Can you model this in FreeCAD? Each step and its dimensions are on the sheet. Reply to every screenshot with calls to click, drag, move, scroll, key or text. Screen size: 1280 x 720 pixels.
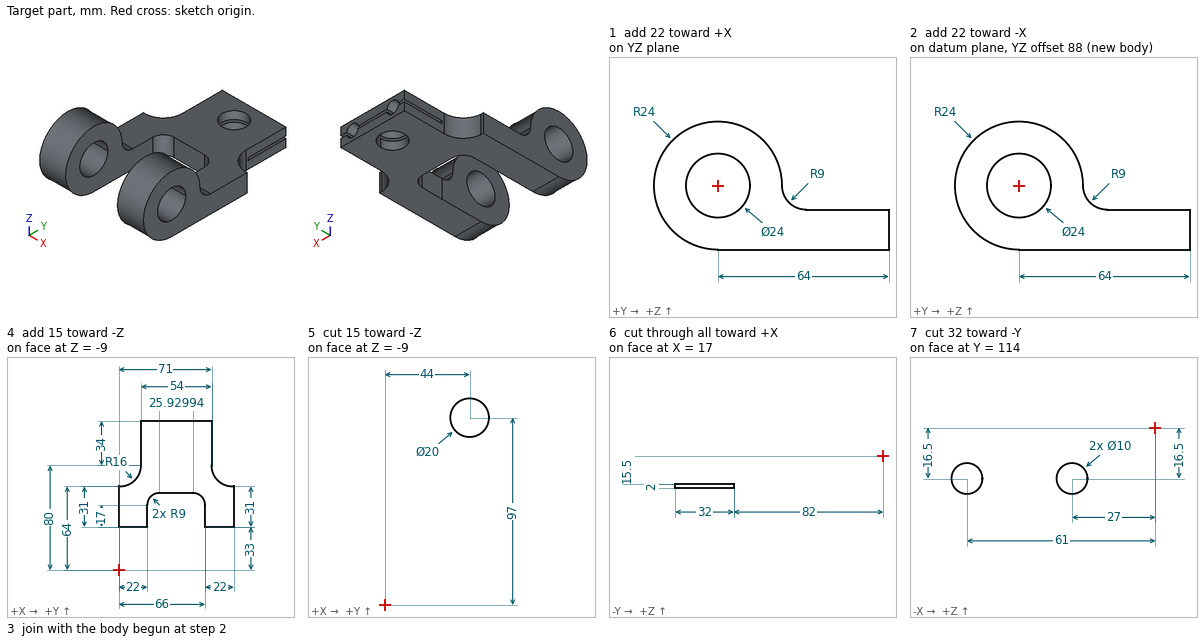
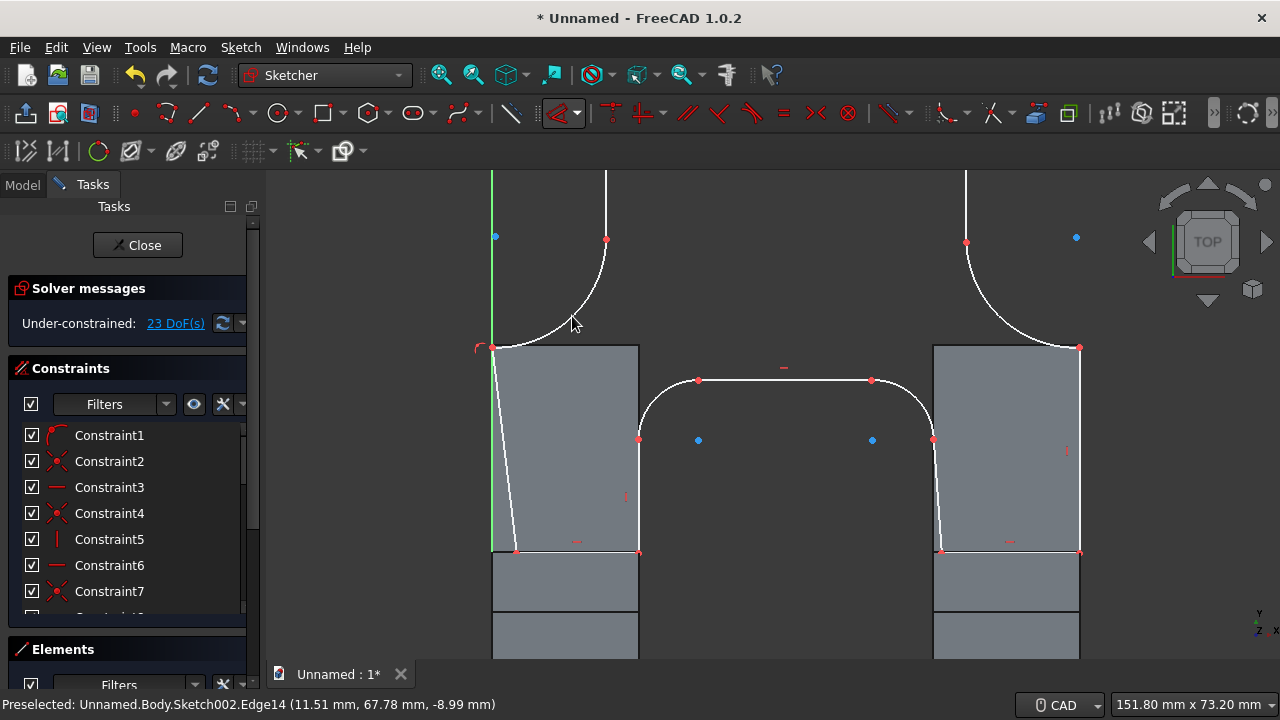
click(639, 519)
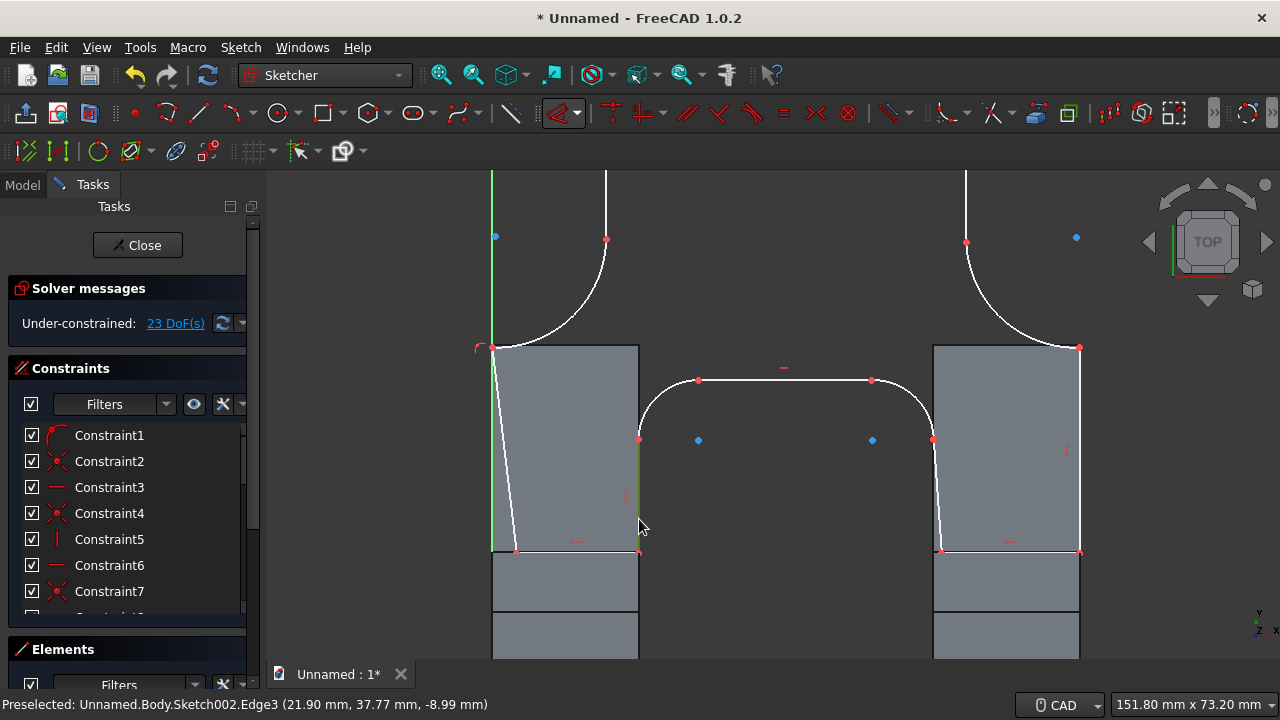
click(671, 387)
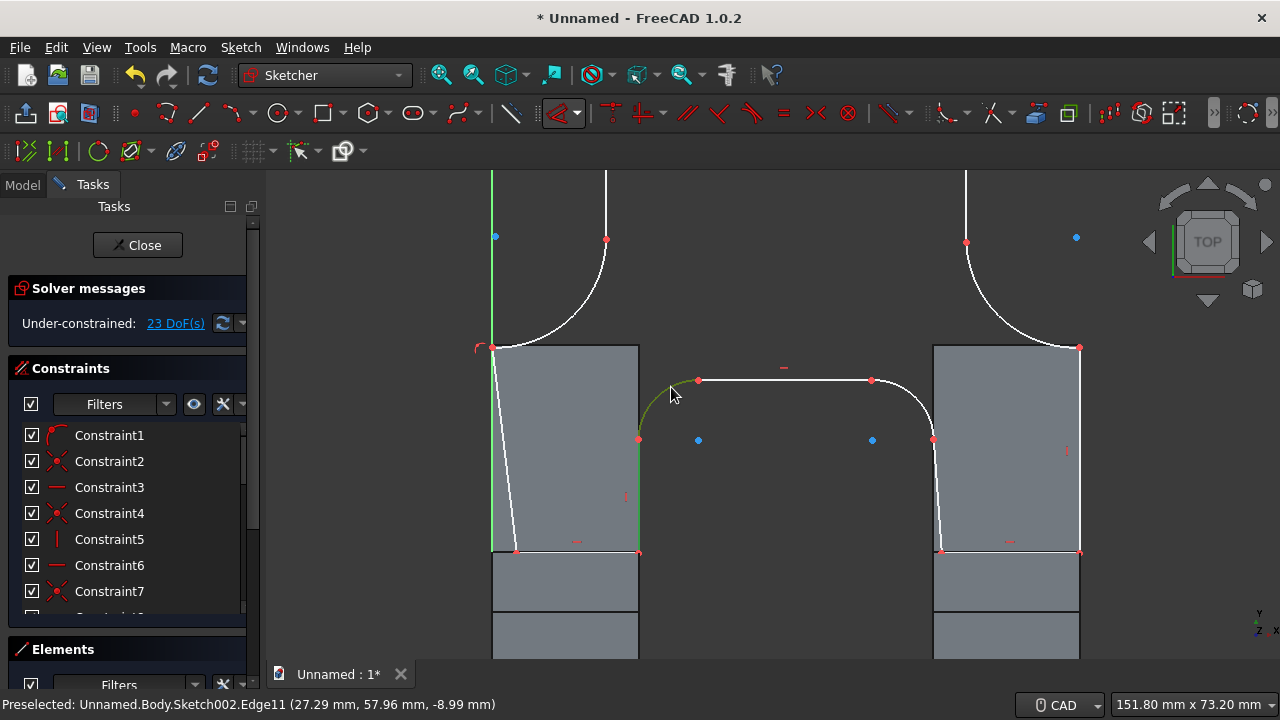
click(752, 114)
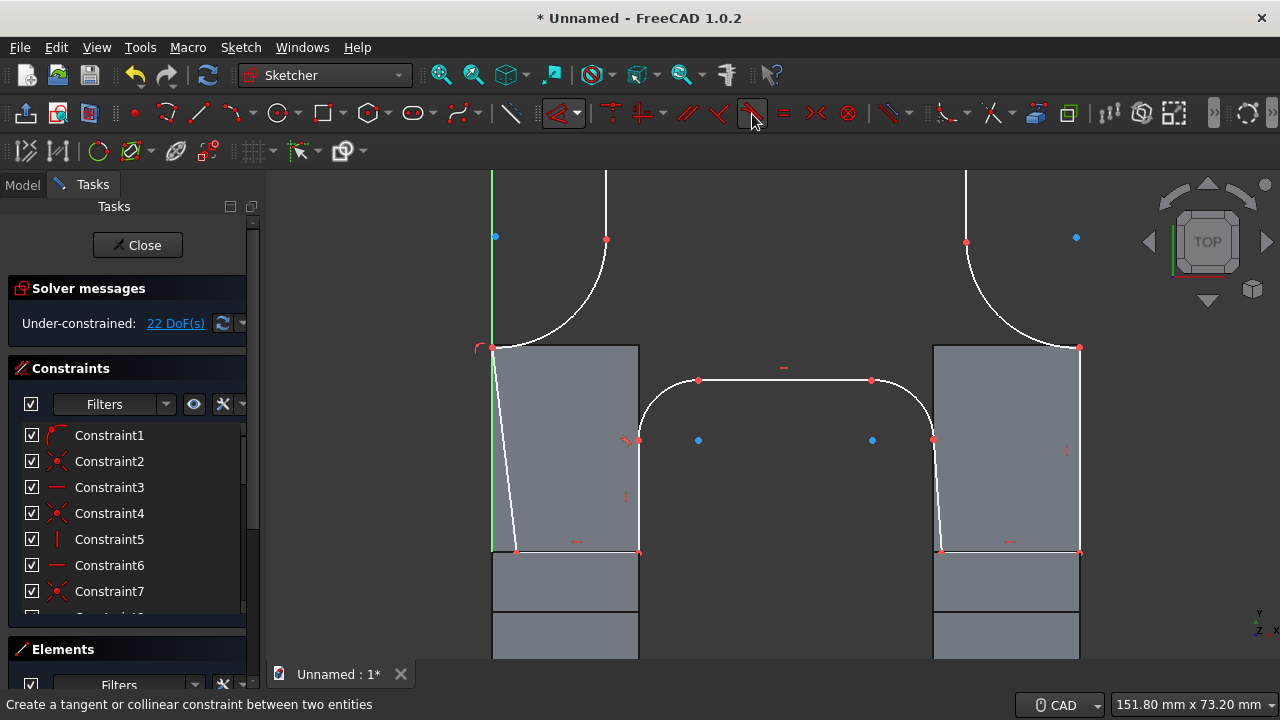
click(750, 380)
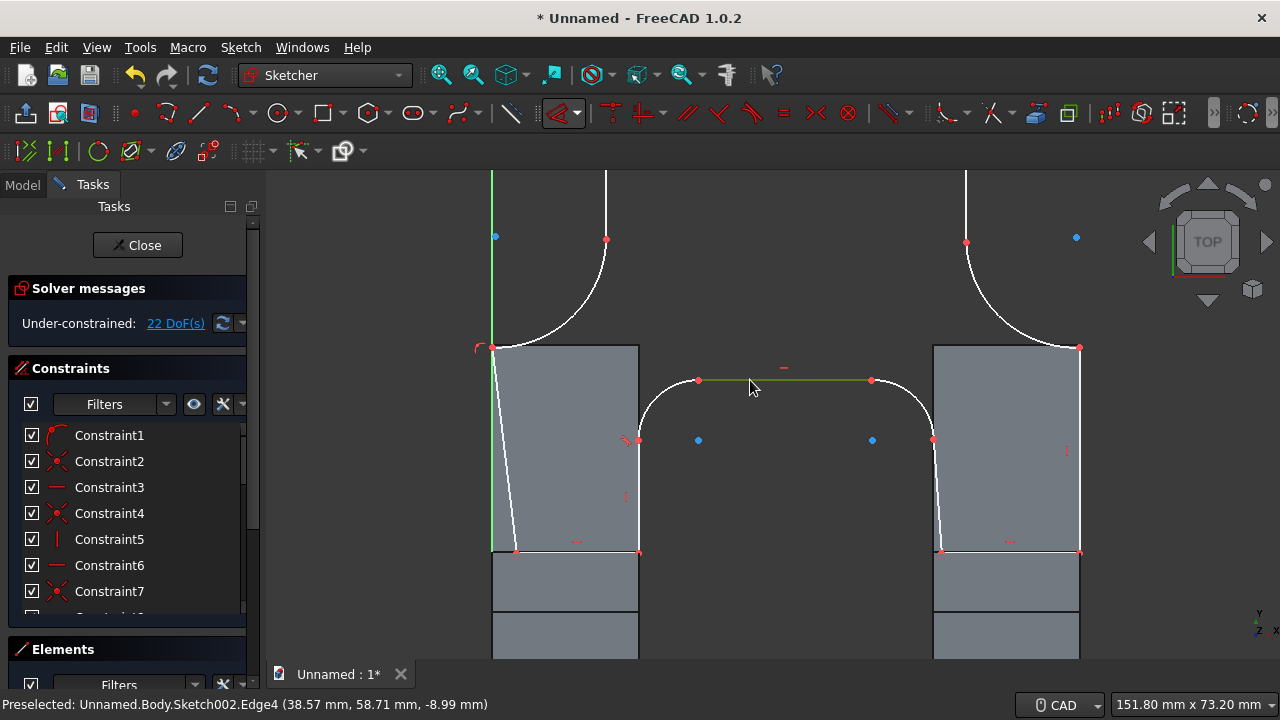
click(671, 387)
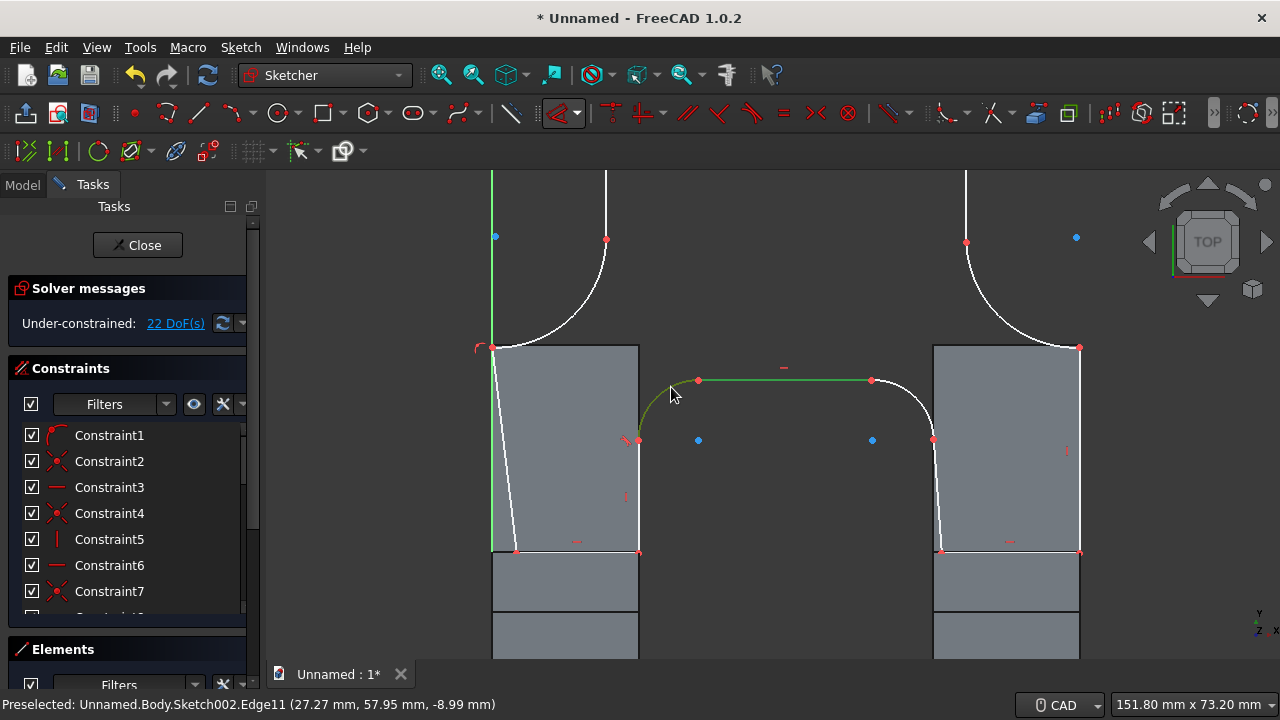
click(752, 114)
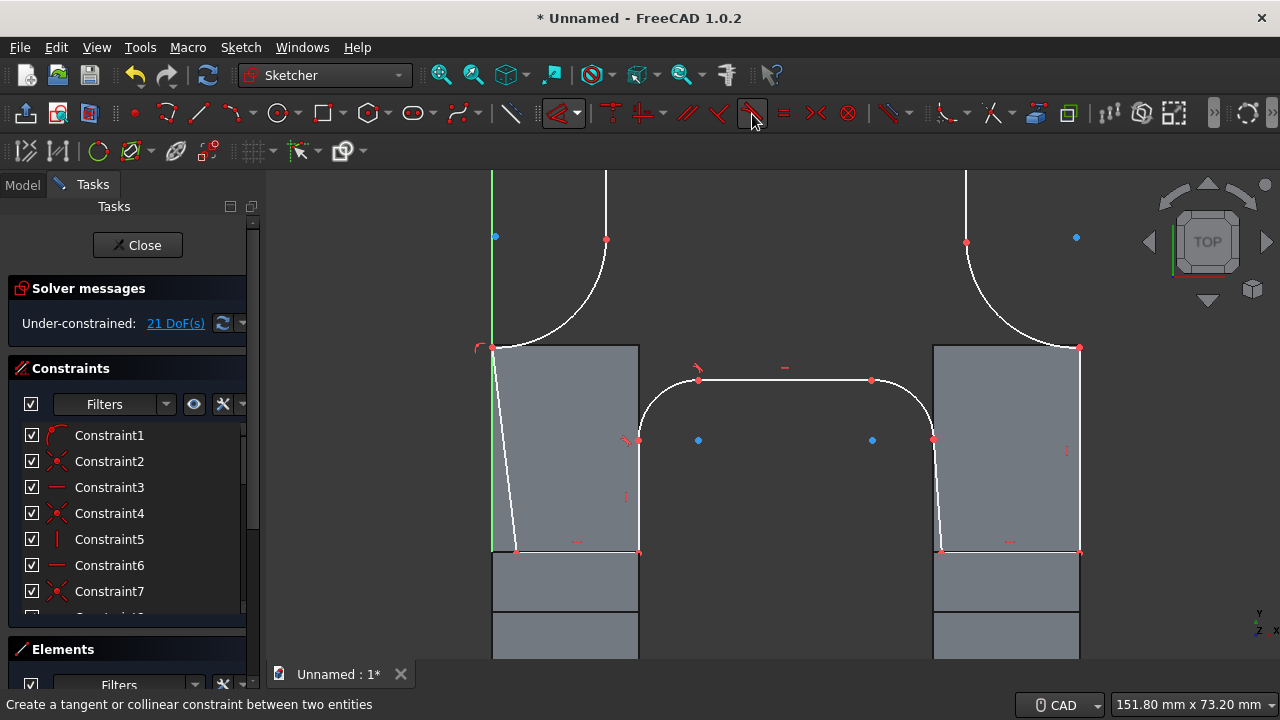
click(751, 380)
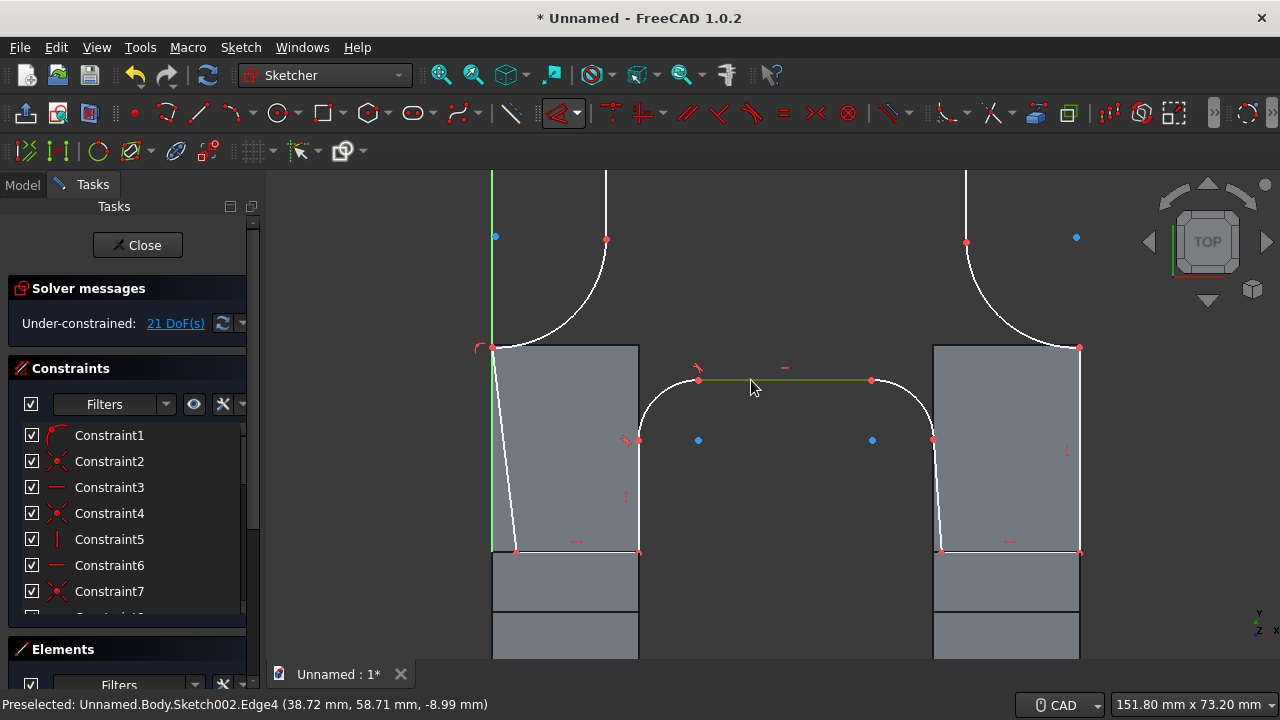
click(927, 412)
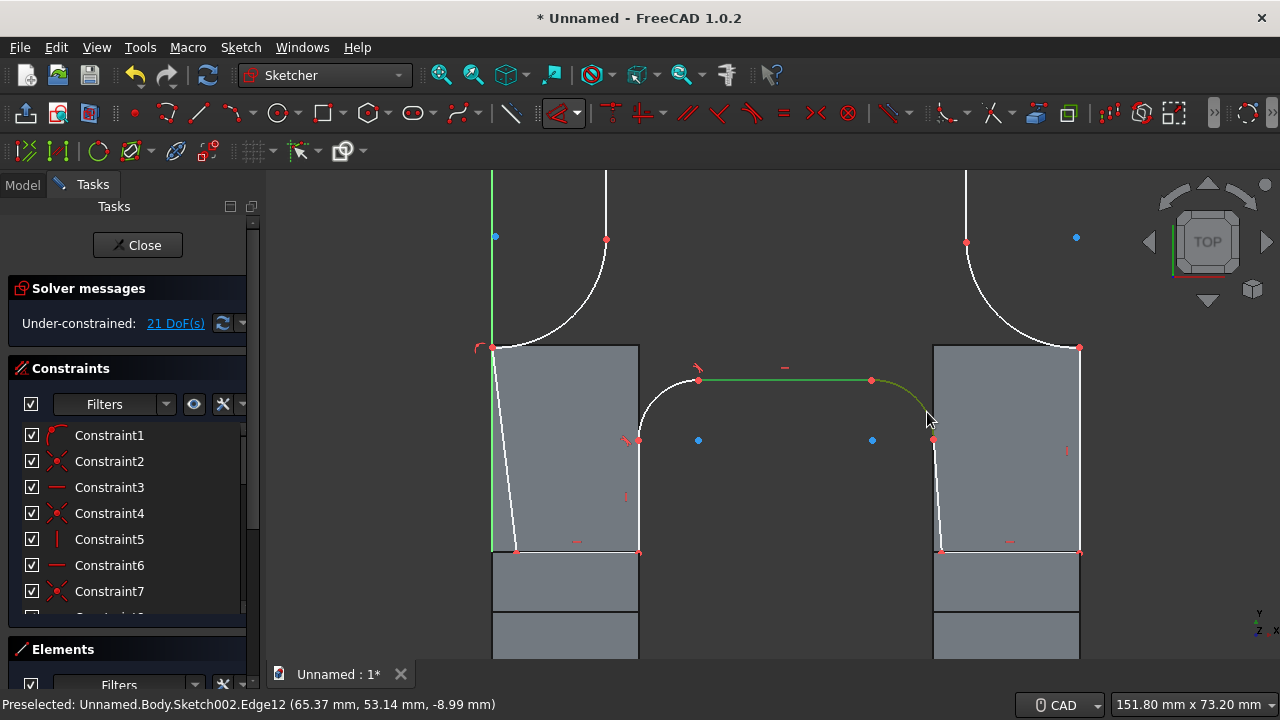
click(752, 114)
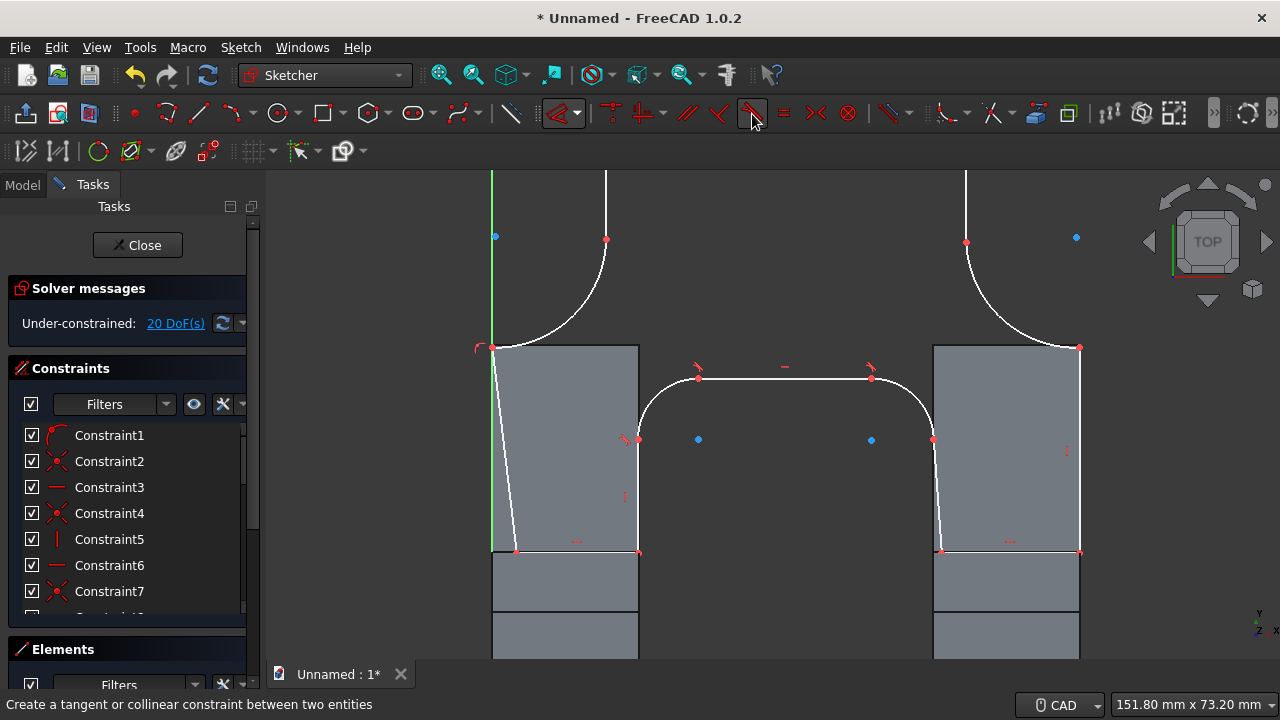
click(936, 474)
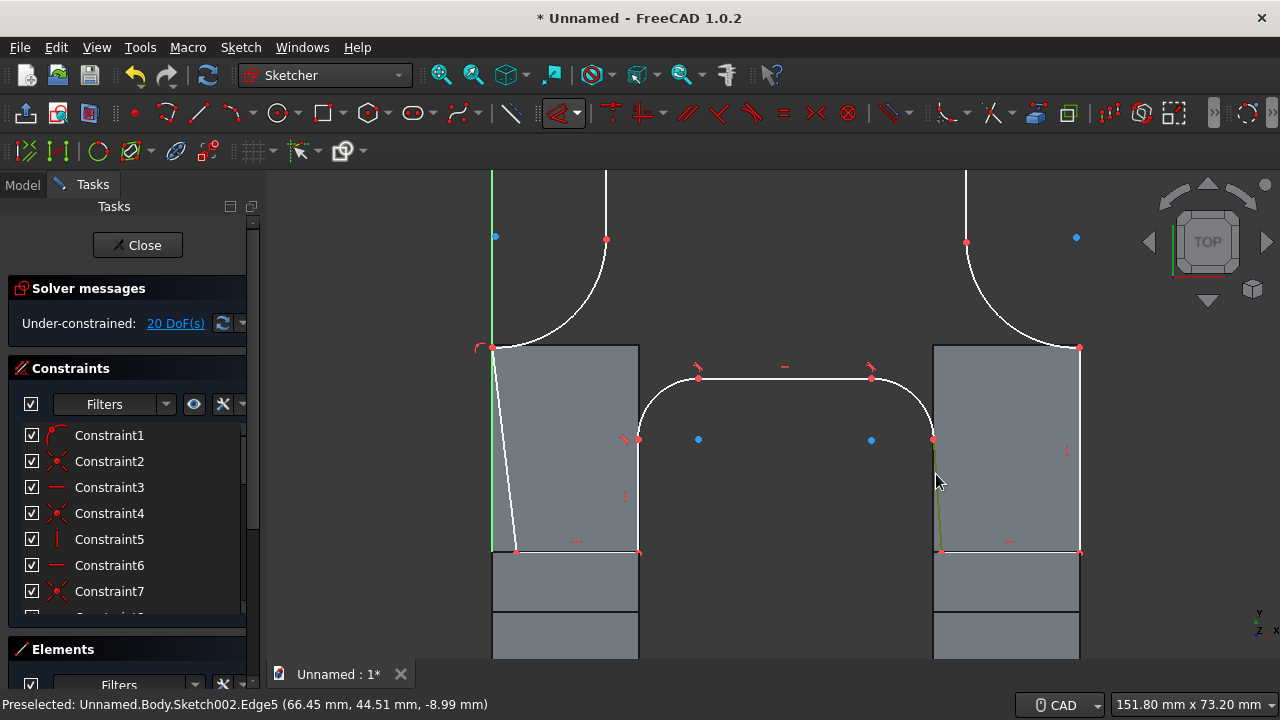
click(927, 412)